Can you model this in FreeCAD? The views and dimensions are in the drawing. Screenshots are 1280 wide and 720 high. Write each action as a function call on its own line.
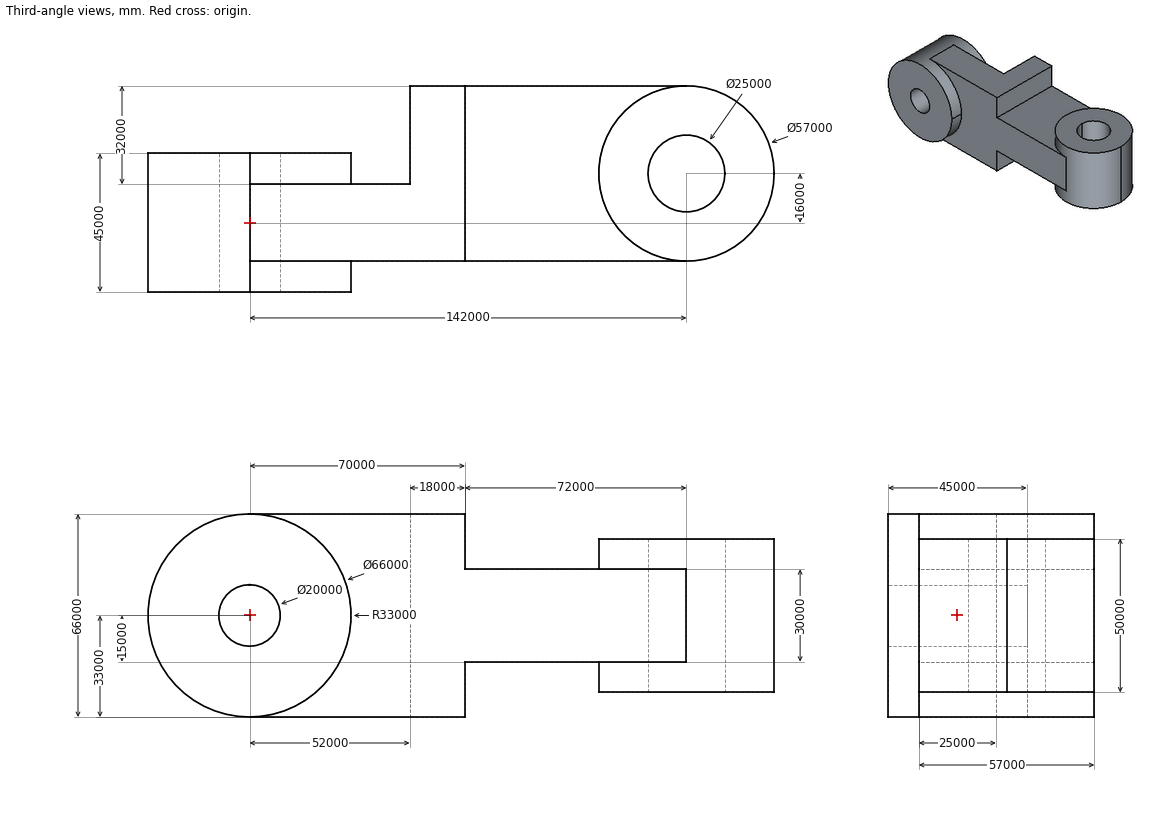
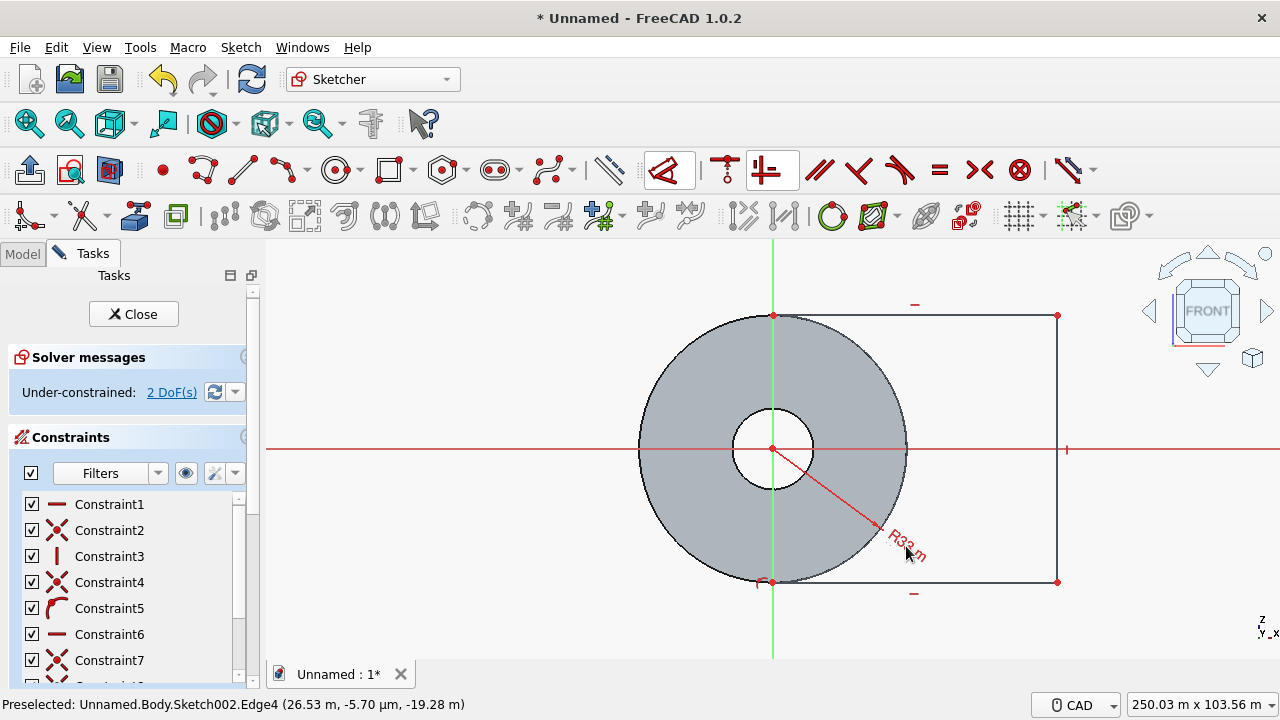
click(773, 315)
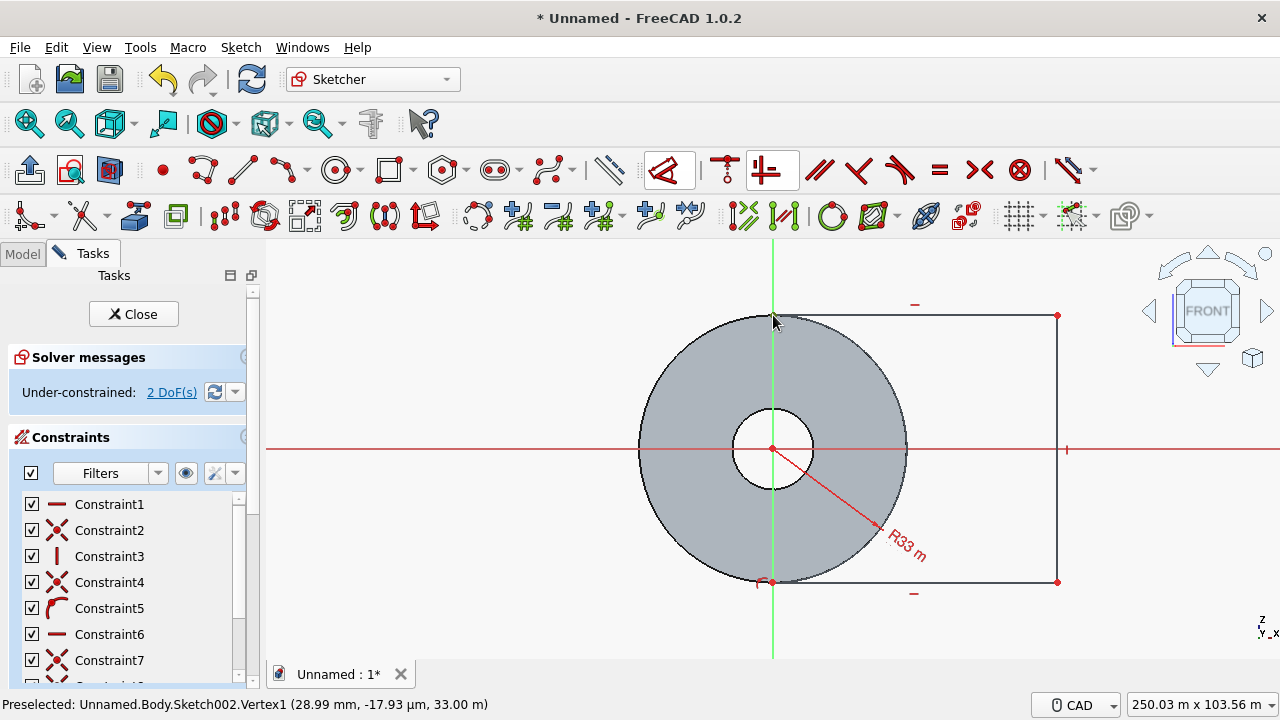
click(773, 527)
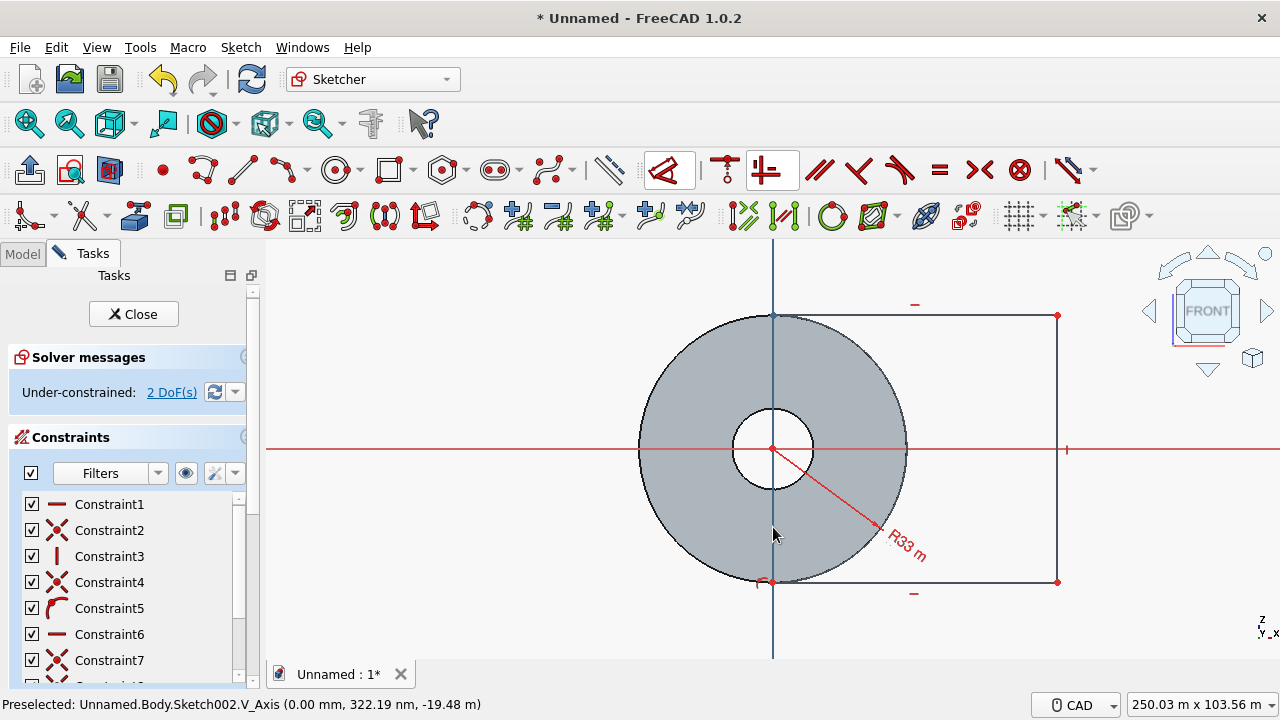
click(726, 170)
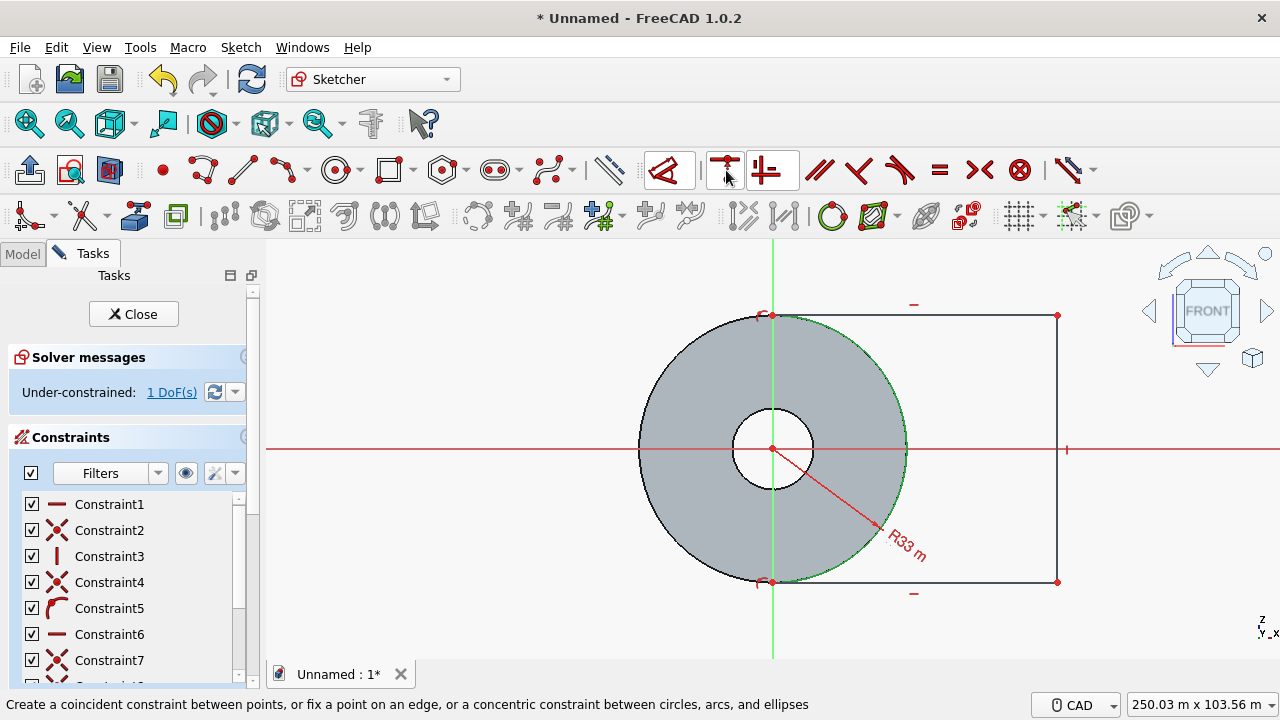
key(d)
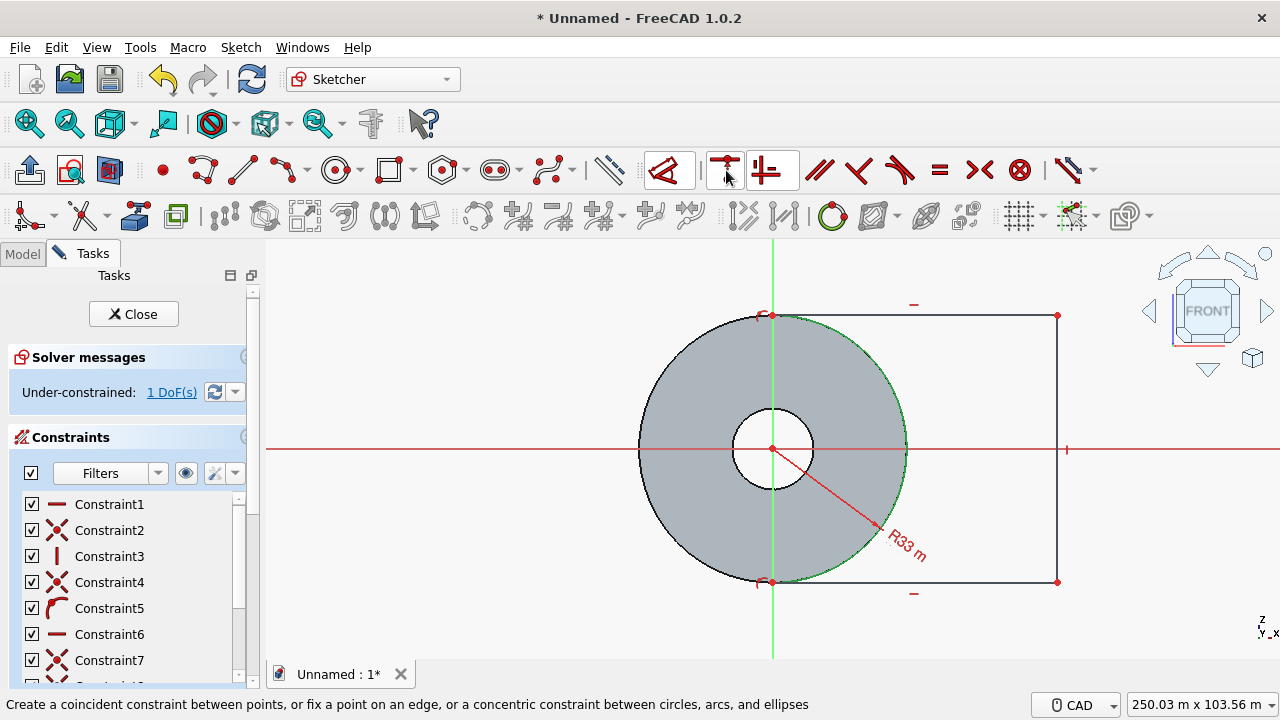
click(858, 315)
click(915, 281)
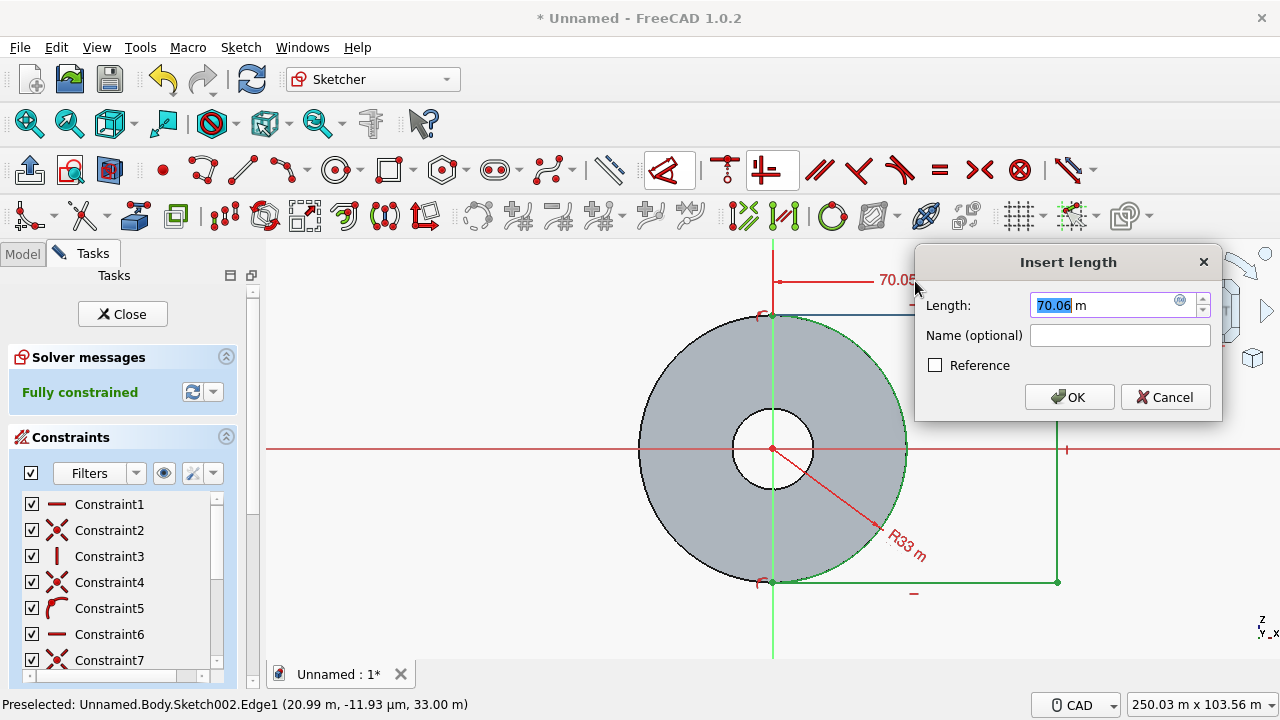
key(ctrl+a)
text(70000 mm)
key(Return)
key(Escape)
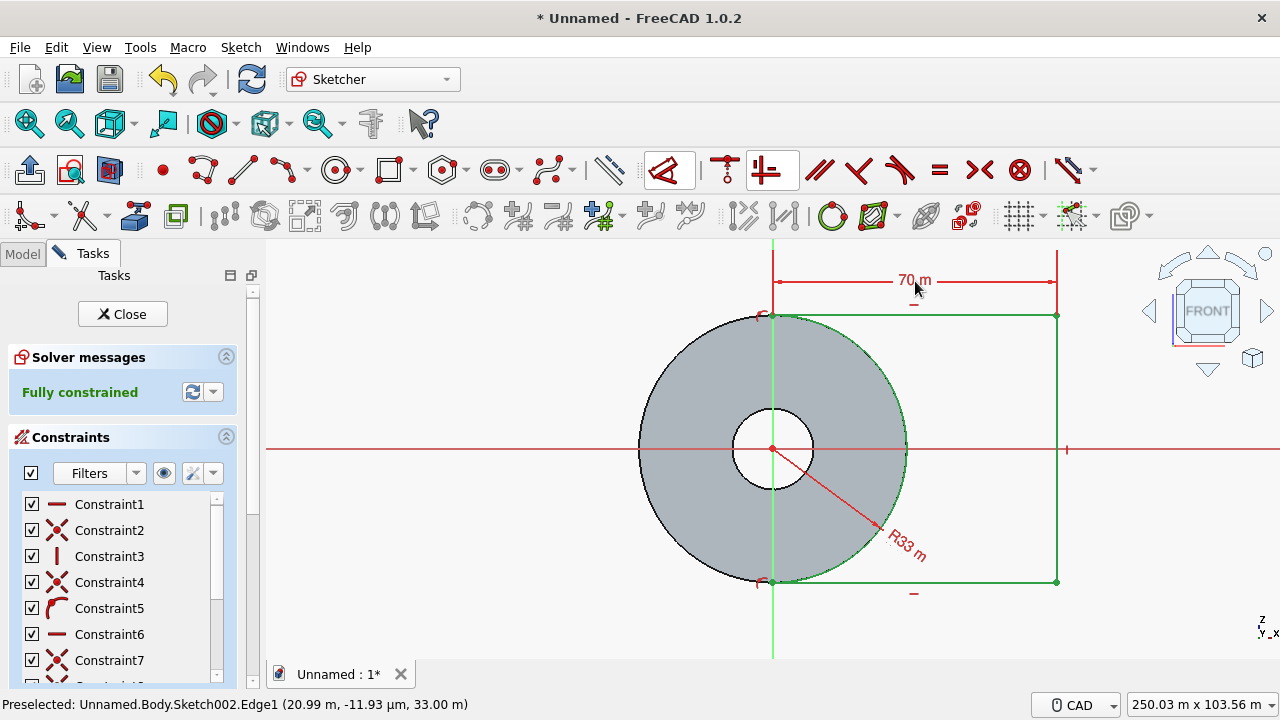
click(123, 314)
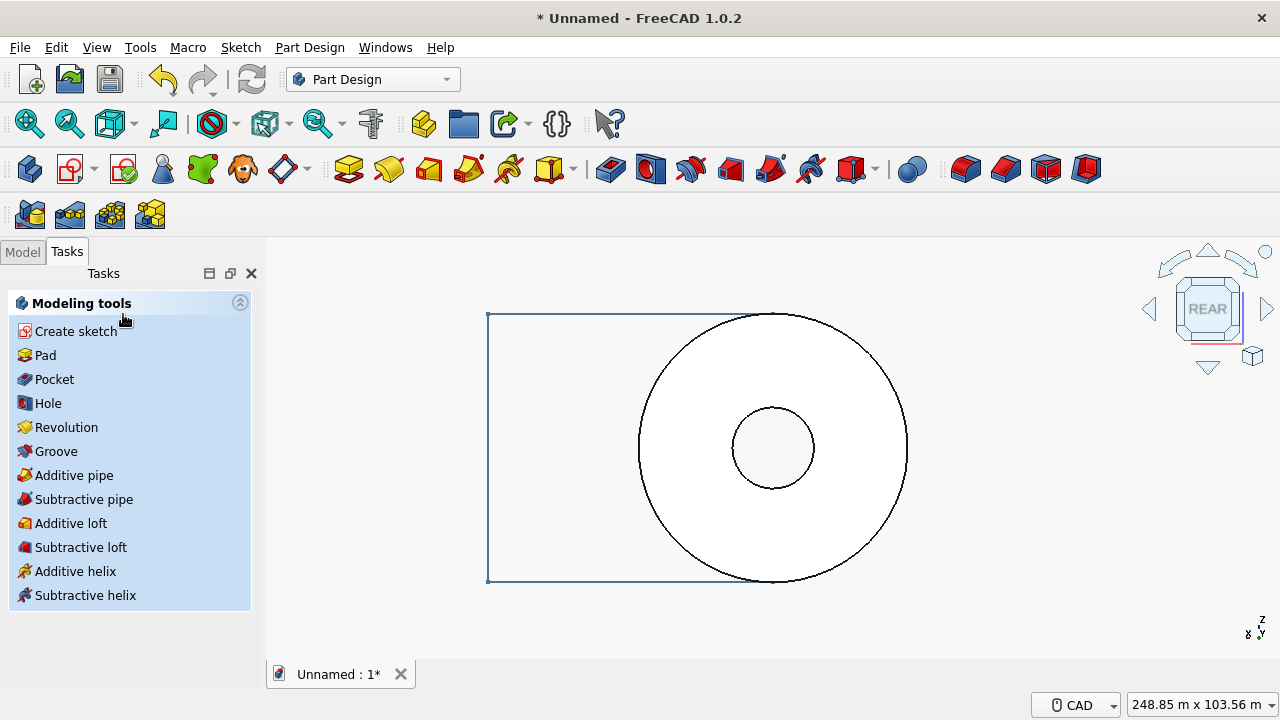
click(350, 170)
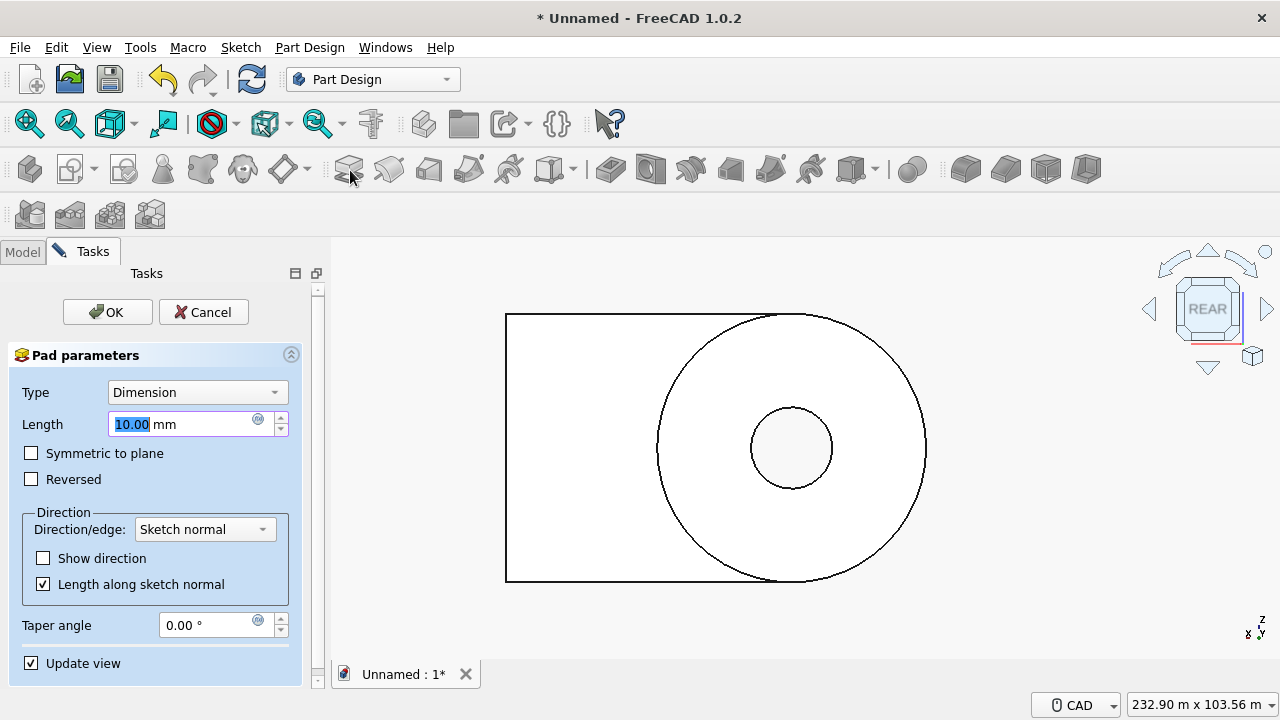
text(25000)
key(Tab)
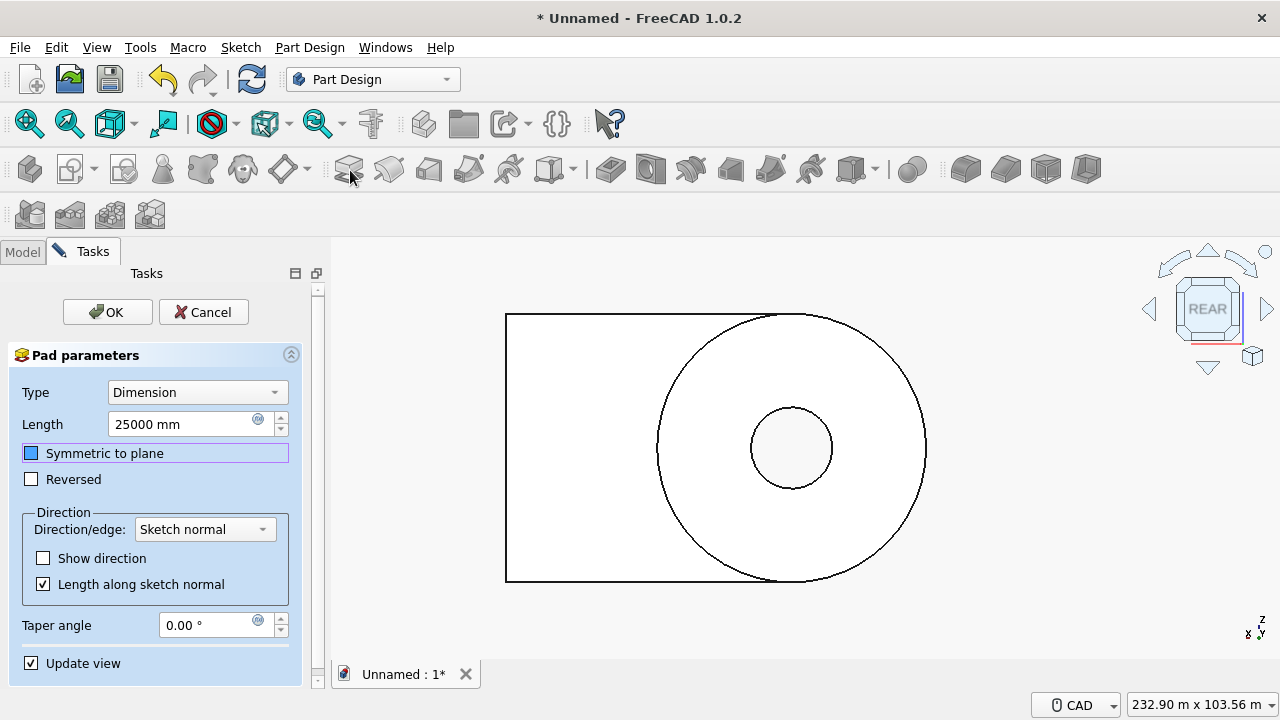
click(30, 453)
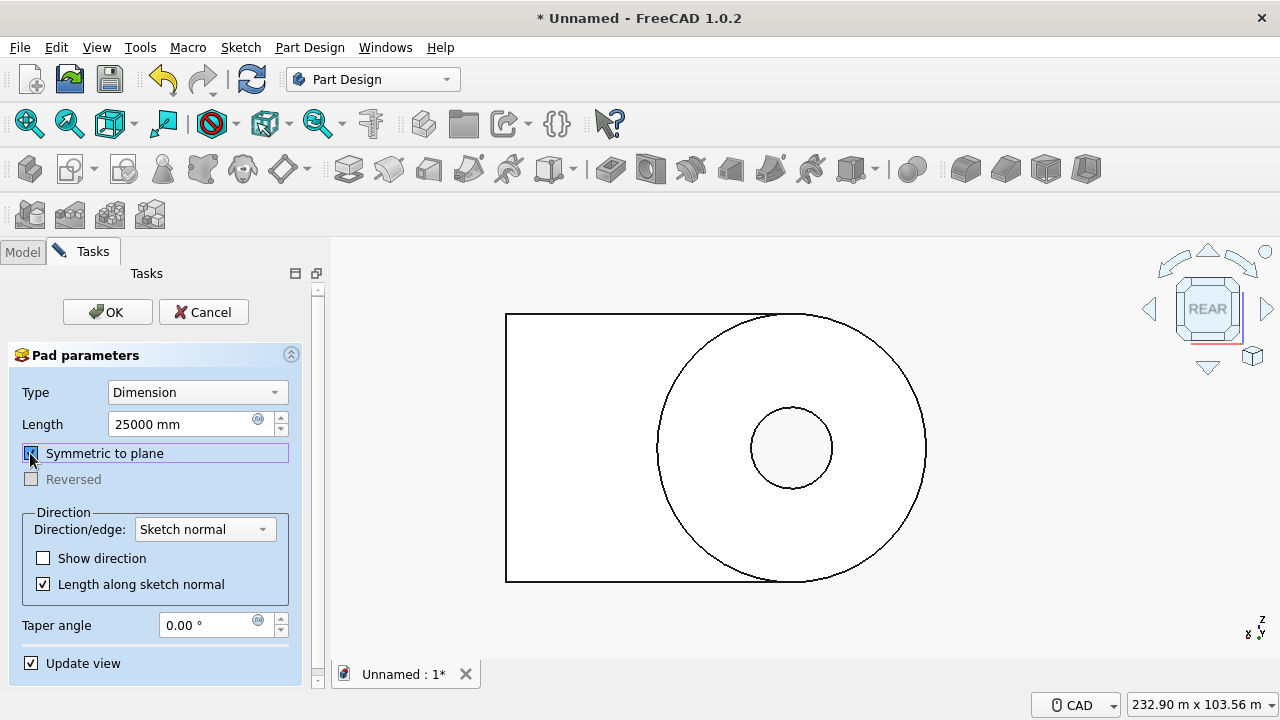
click(108, 312)